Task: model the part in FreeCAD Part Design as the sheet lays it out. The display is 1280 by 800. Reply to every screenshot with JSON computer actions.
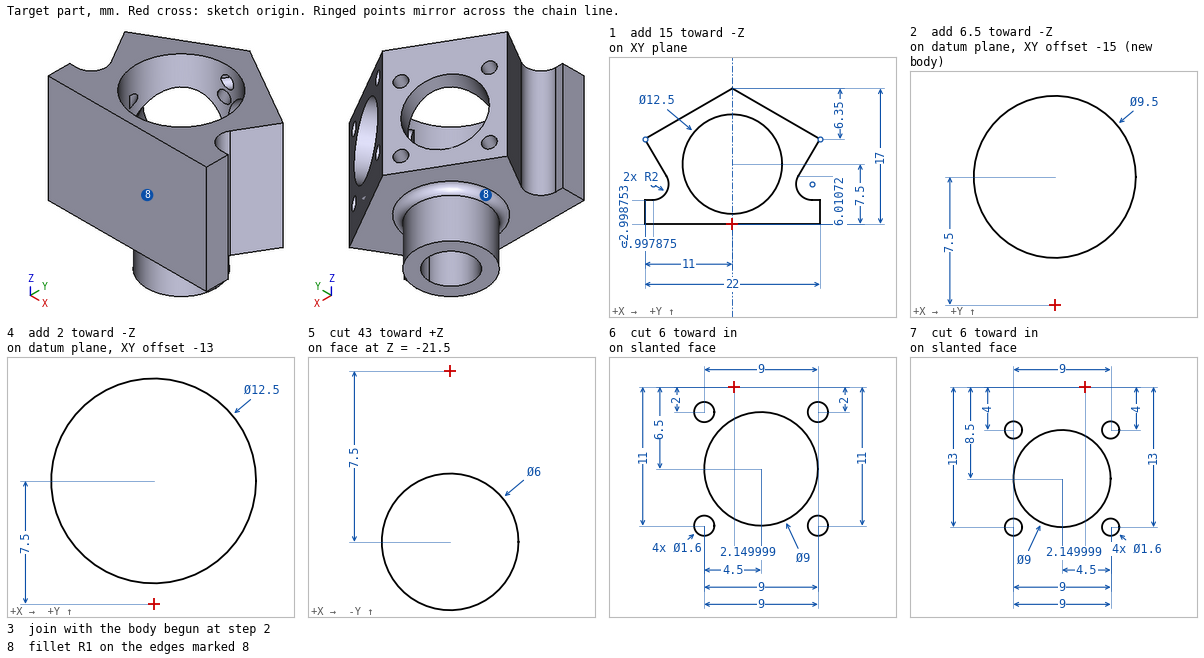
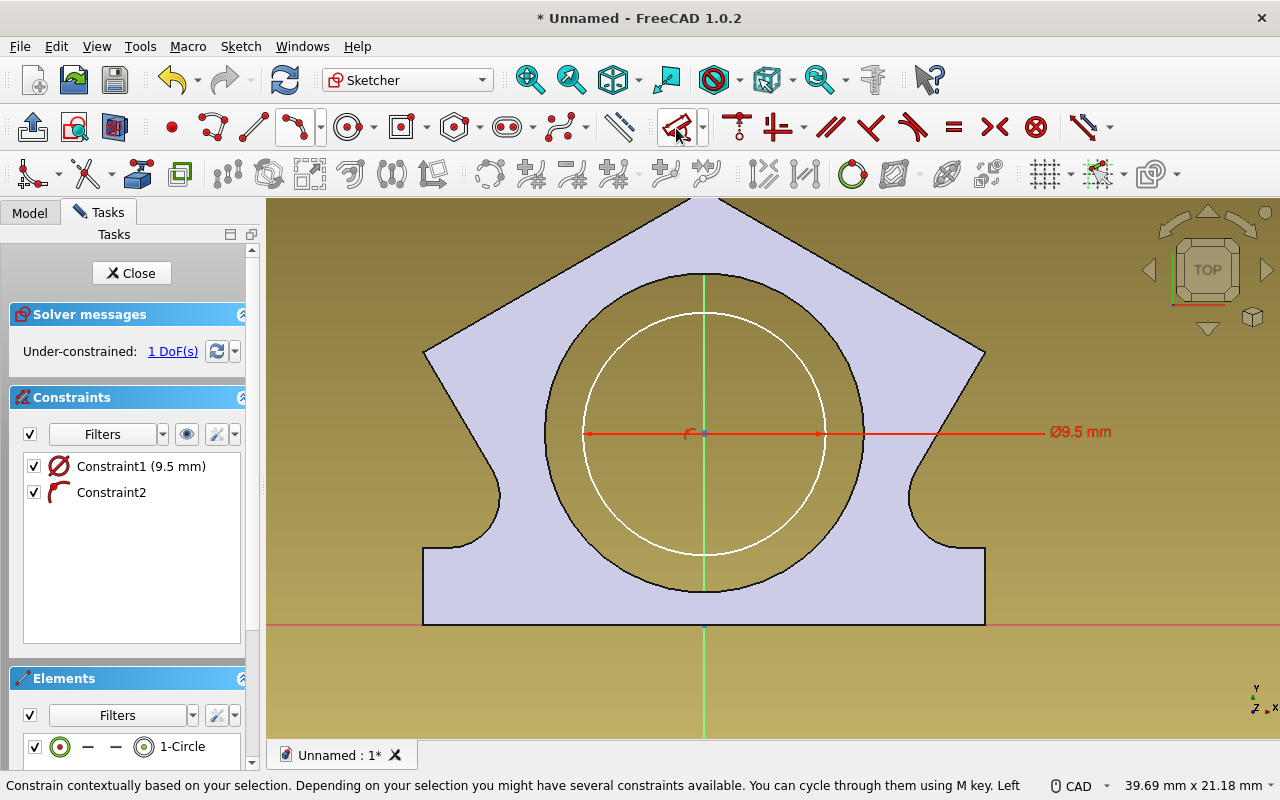
{"action": "left_click", "coordinate": [704, 434]}
{"action": "left_click", "coordinate": [738, 529]}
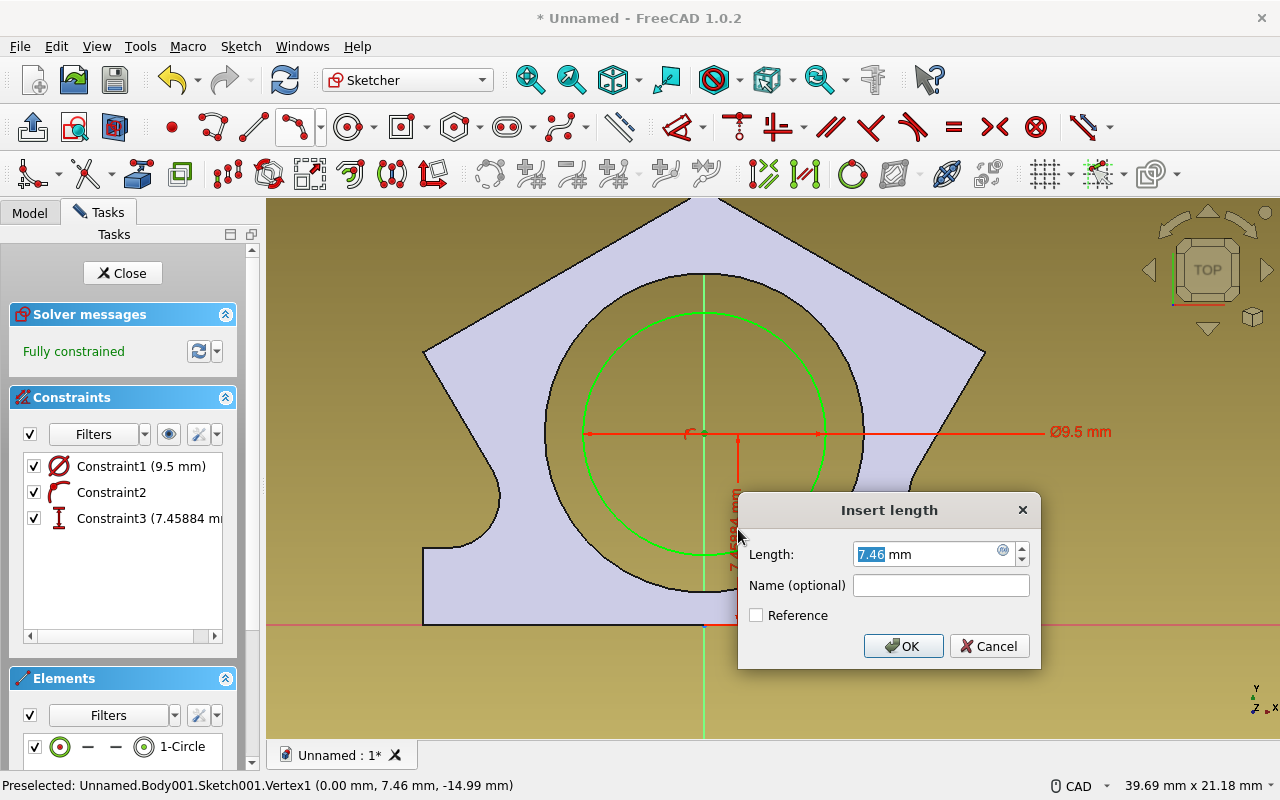
{"action": "type", "text": "7.5"}
{"action": "key", "text": "Return"}
{"action": "key", "text": "Escape"}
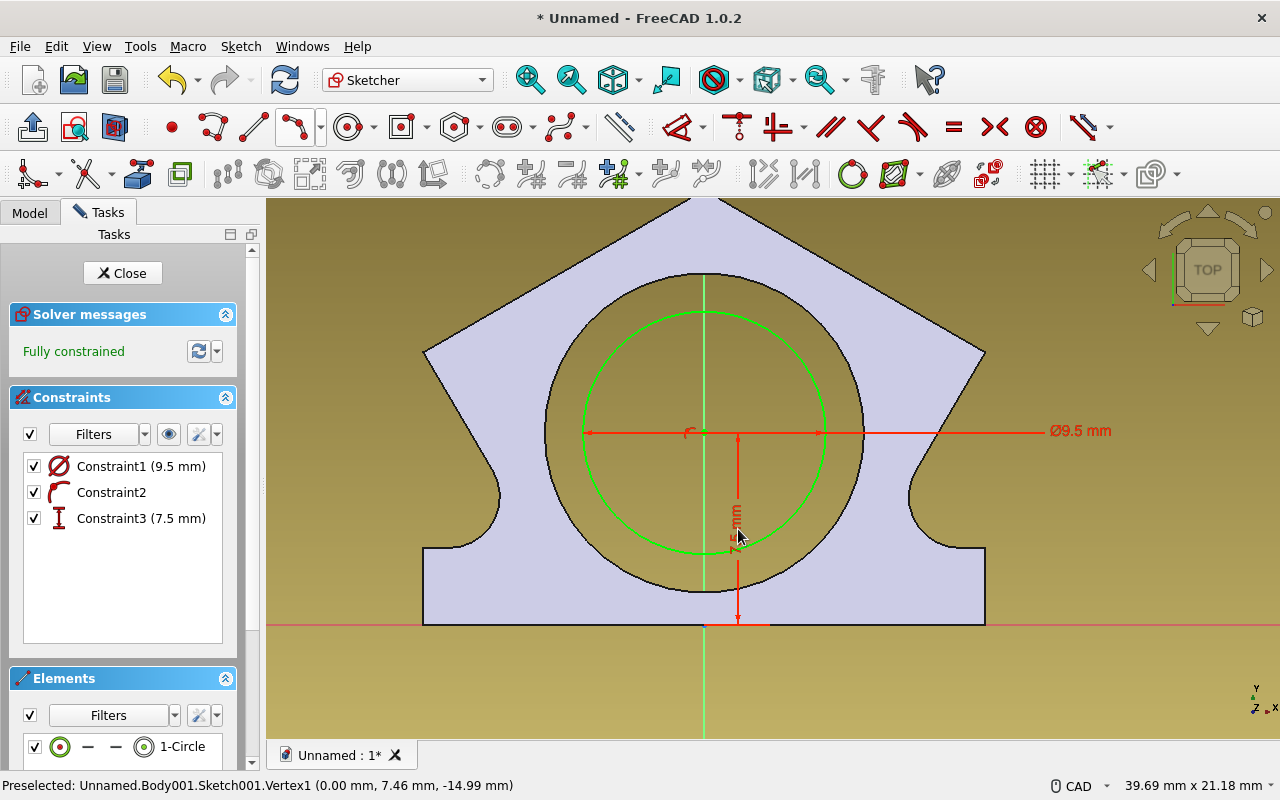
{"action": "left_click", "coordinate": [123, 273]}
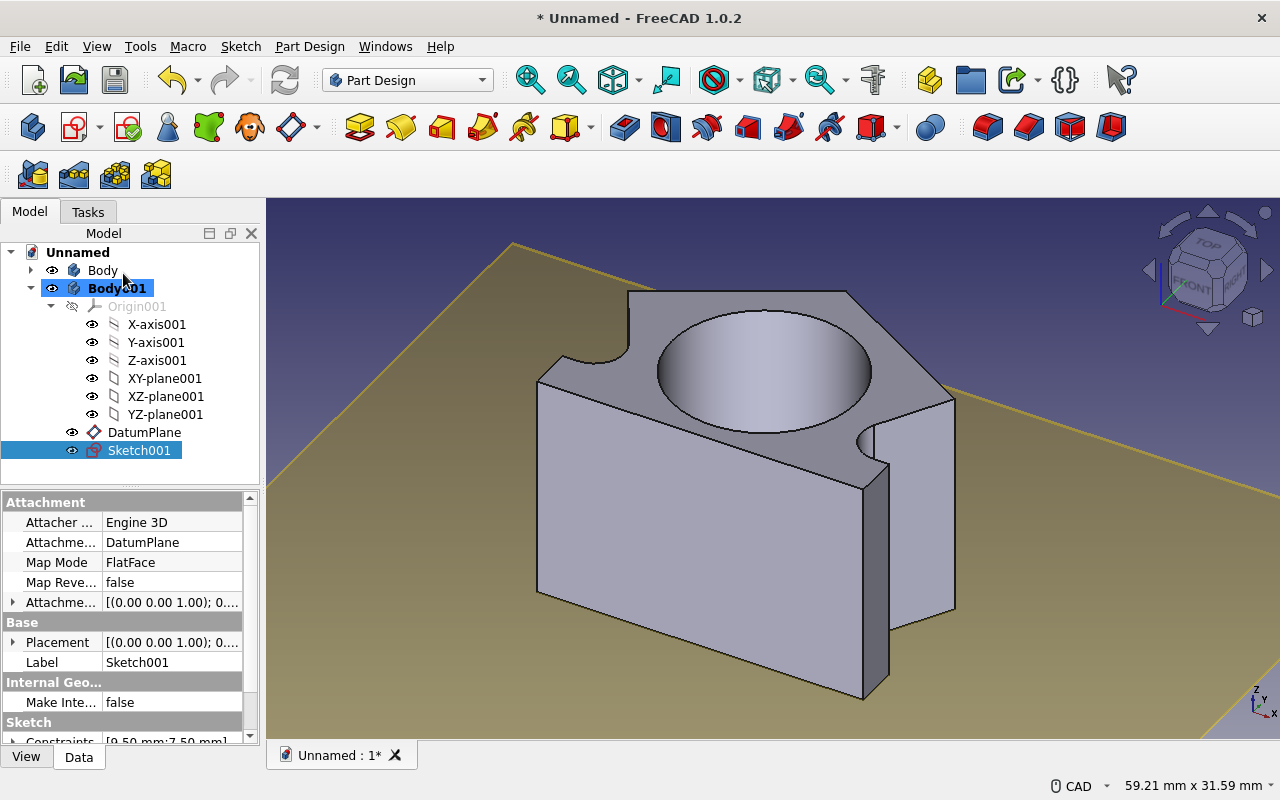
{"action": "left_click", "coordinate": [360, 128]}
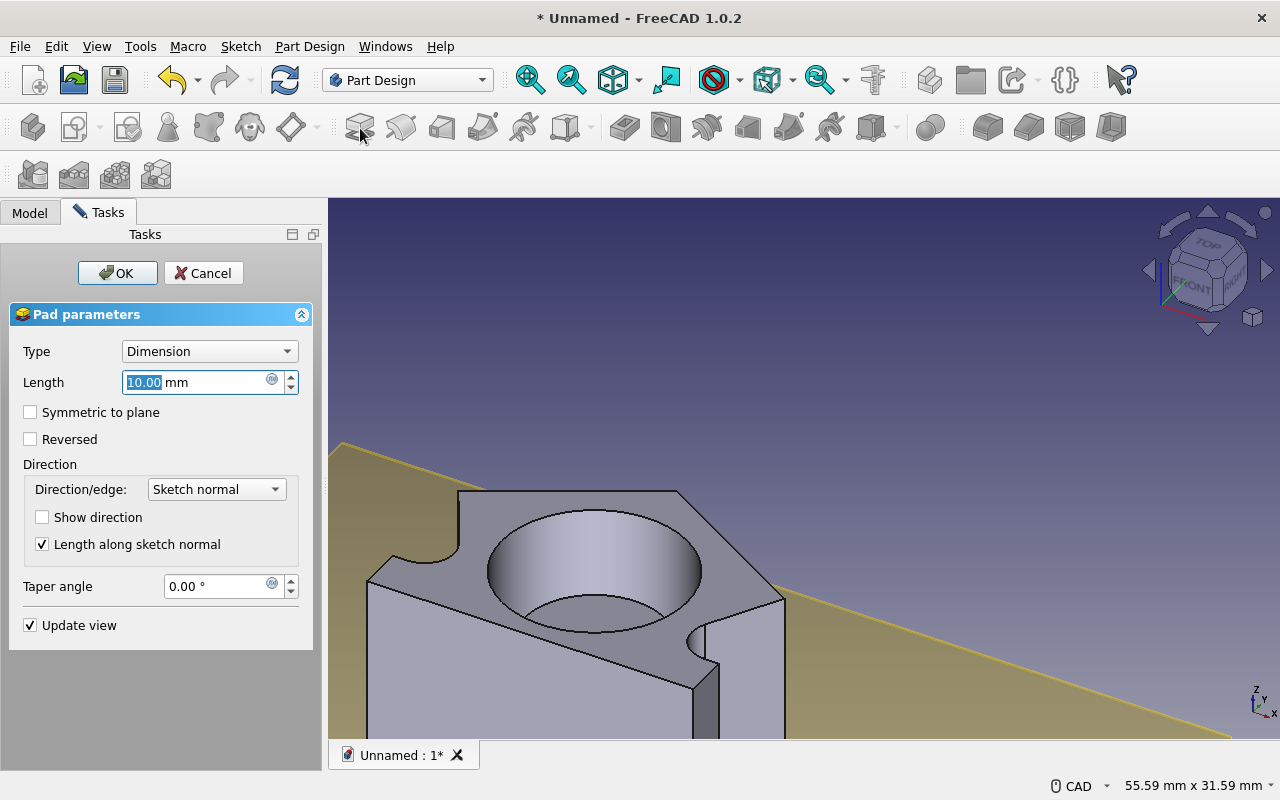
{"action": "type", "text": "6.5"}
{"action": "key", "text": "Tab"}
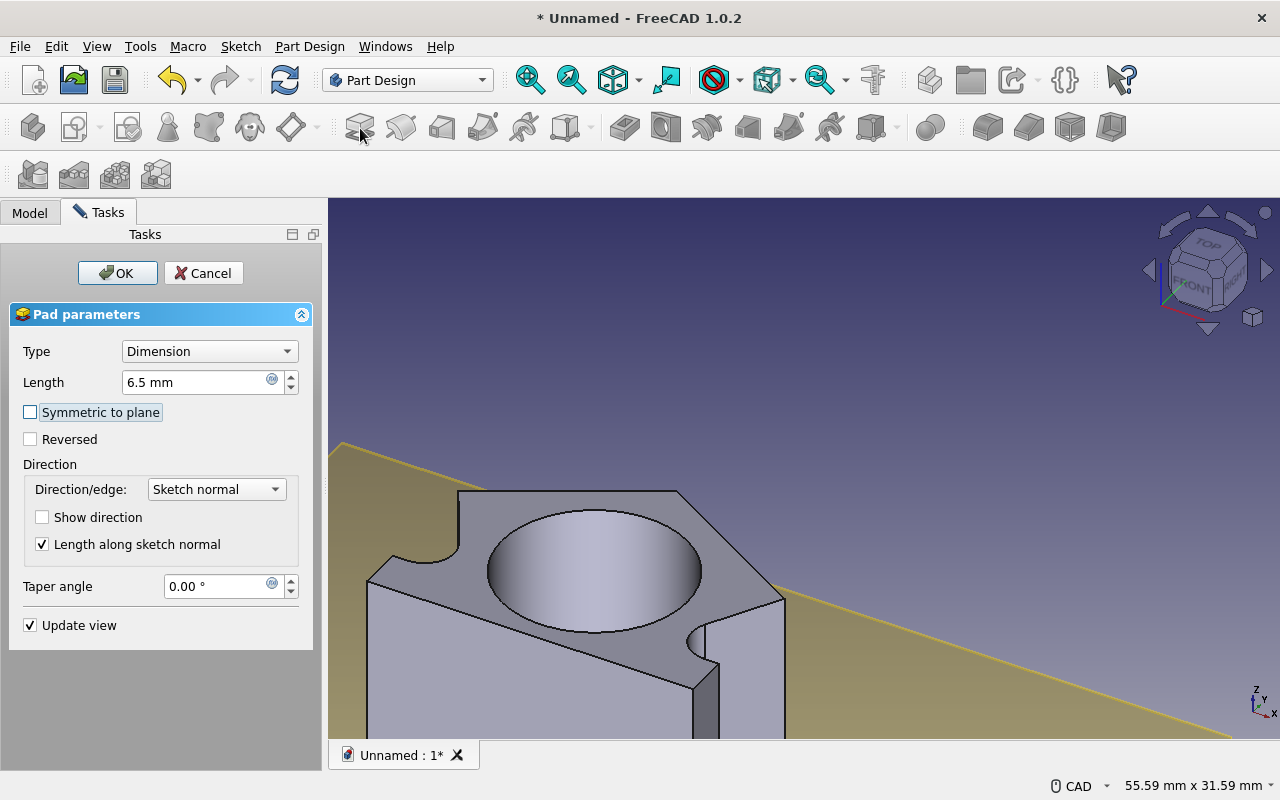
{"action": "left_click", "coordinate": [31, 439]}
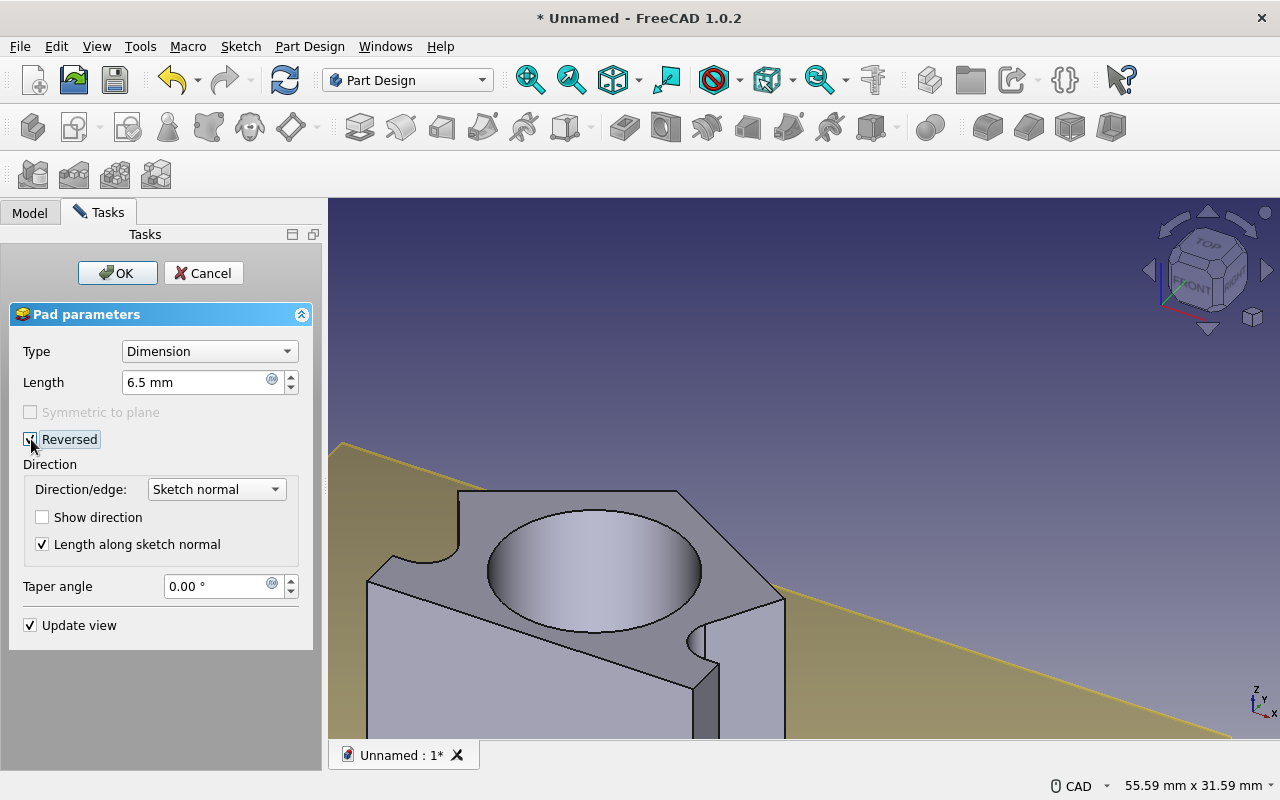
{"action": "left_click", "coordinate": [118, 273]}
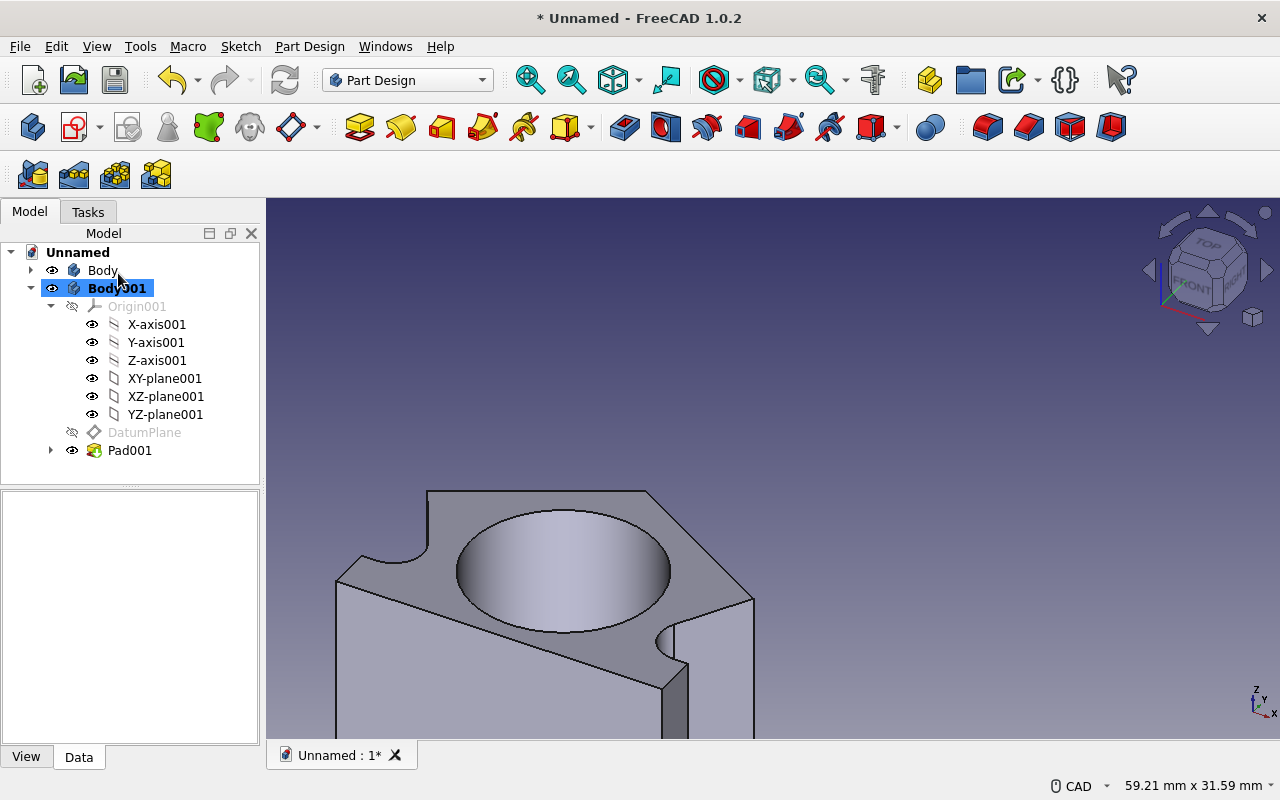
{"action": "left_click", "coordinate": [531, 80]}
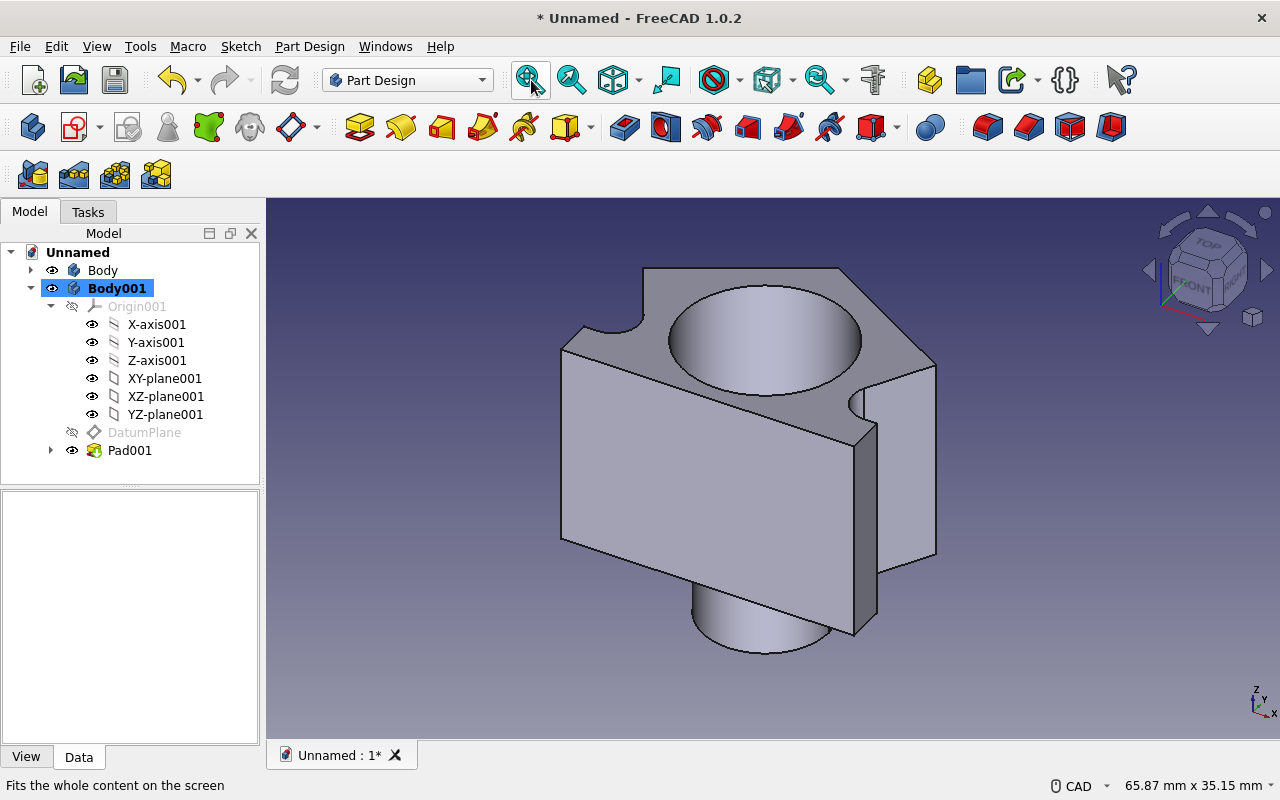
{"action": "double_click", "coordinate": [97, 270]}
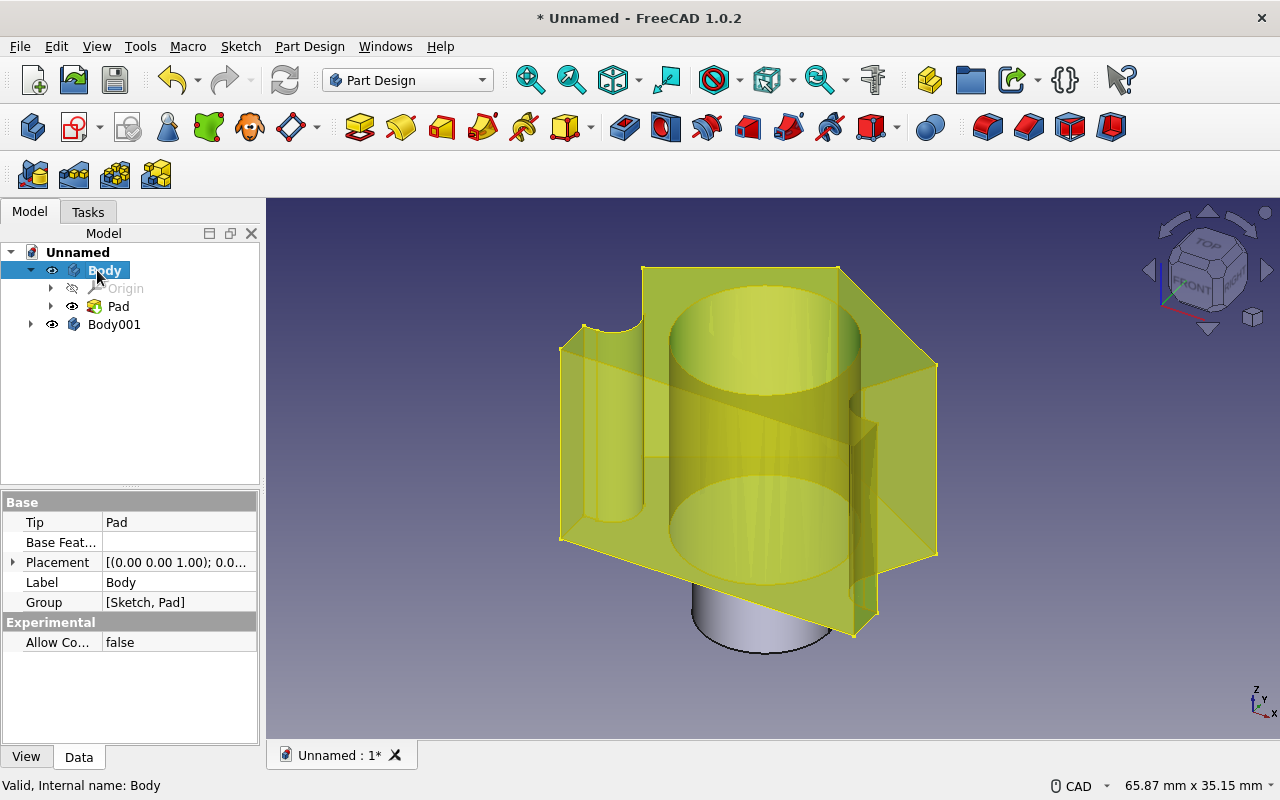
{"action": "left_click", "coordinate": [97, 270]}